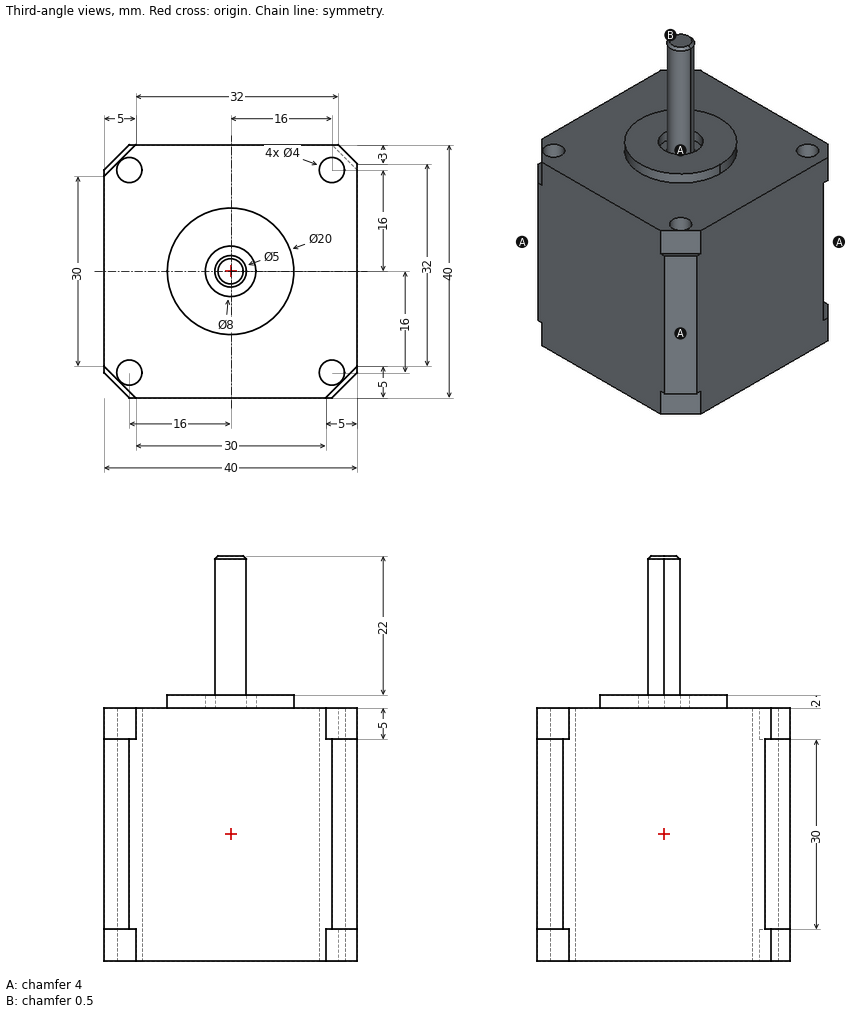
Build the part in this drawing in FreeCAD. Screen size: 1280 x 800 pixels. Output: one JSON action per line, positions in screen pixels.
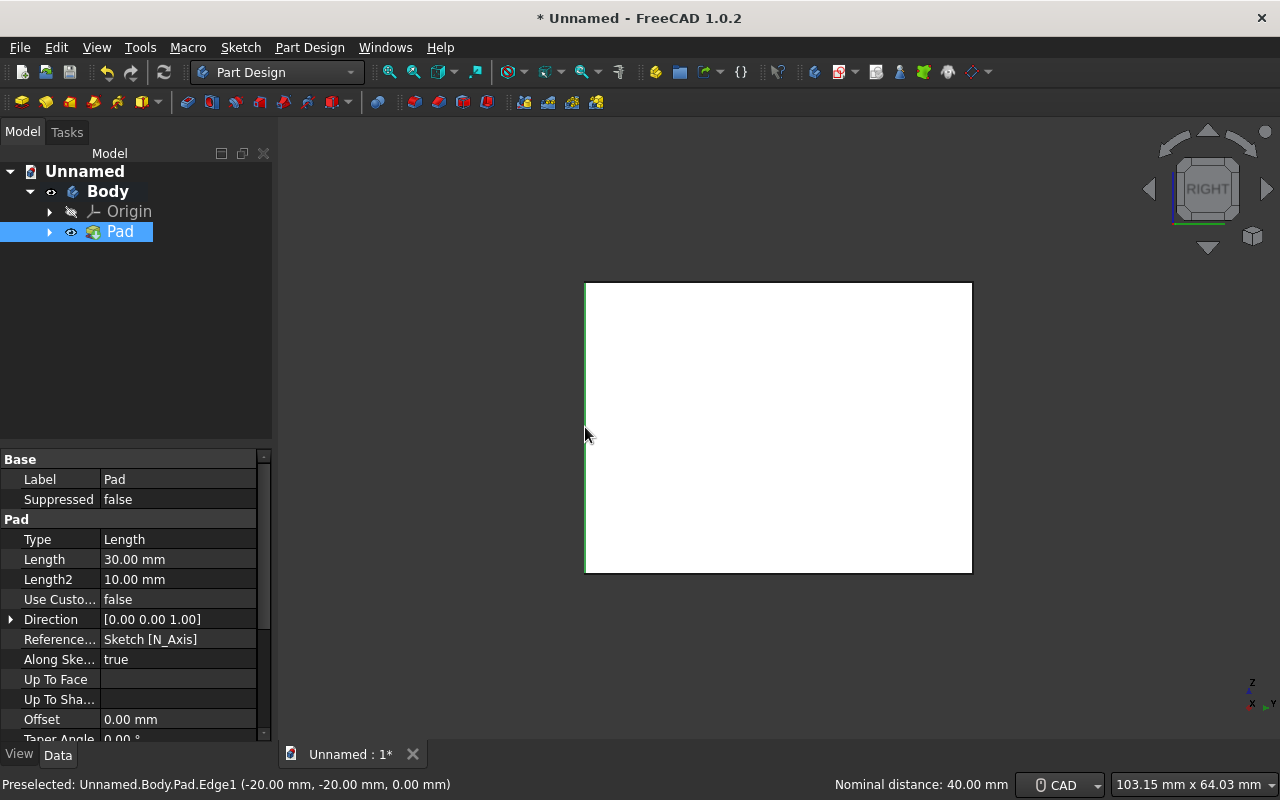
{"action": "left_click", "coordinate": [973, 427], "text": "ctrl"}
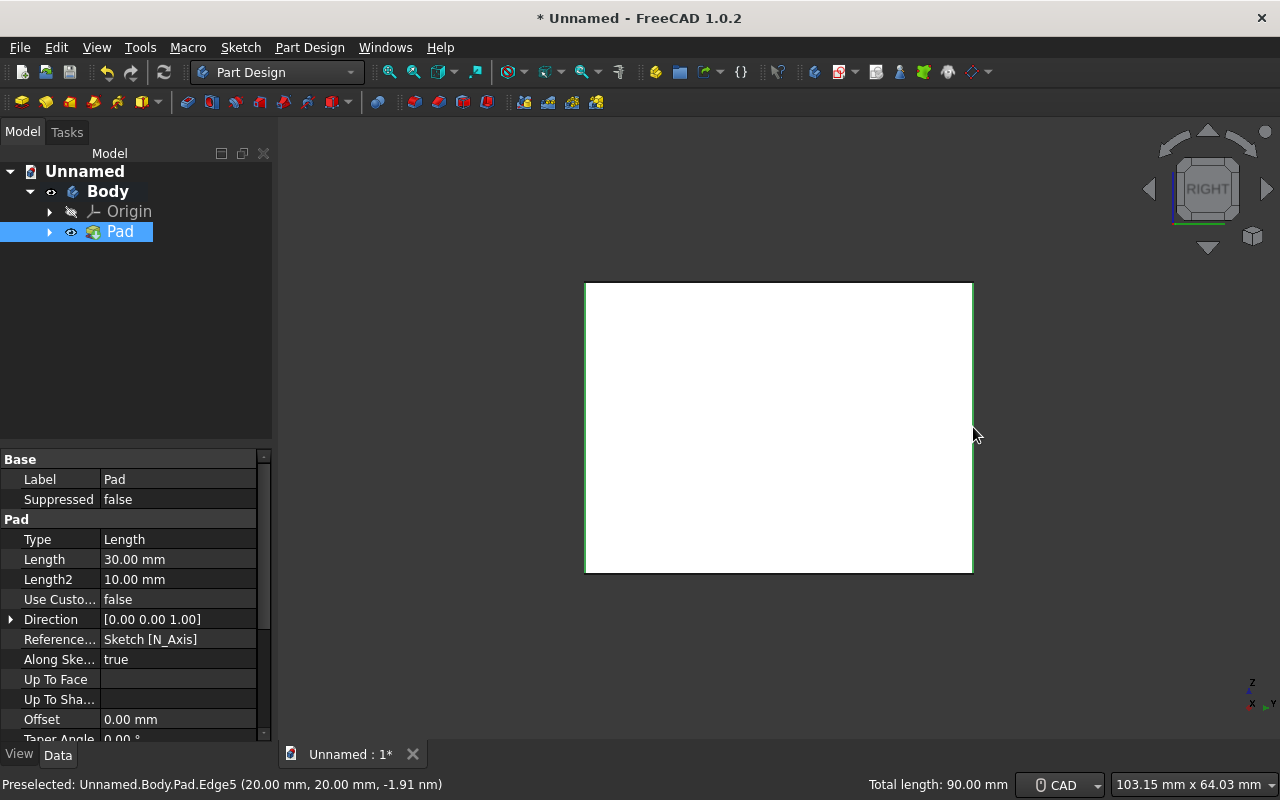
{"action": "key", "text": "5"}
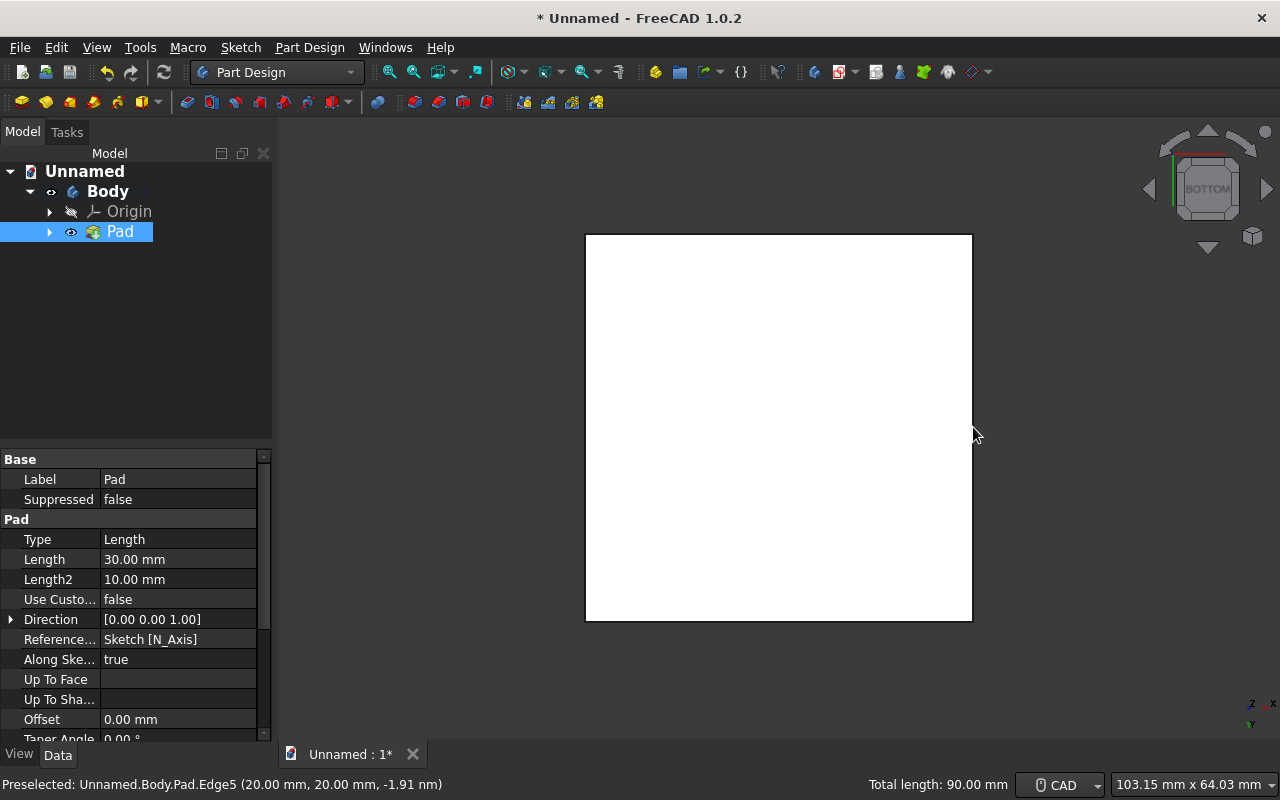
{"action": "key", "text": "4"}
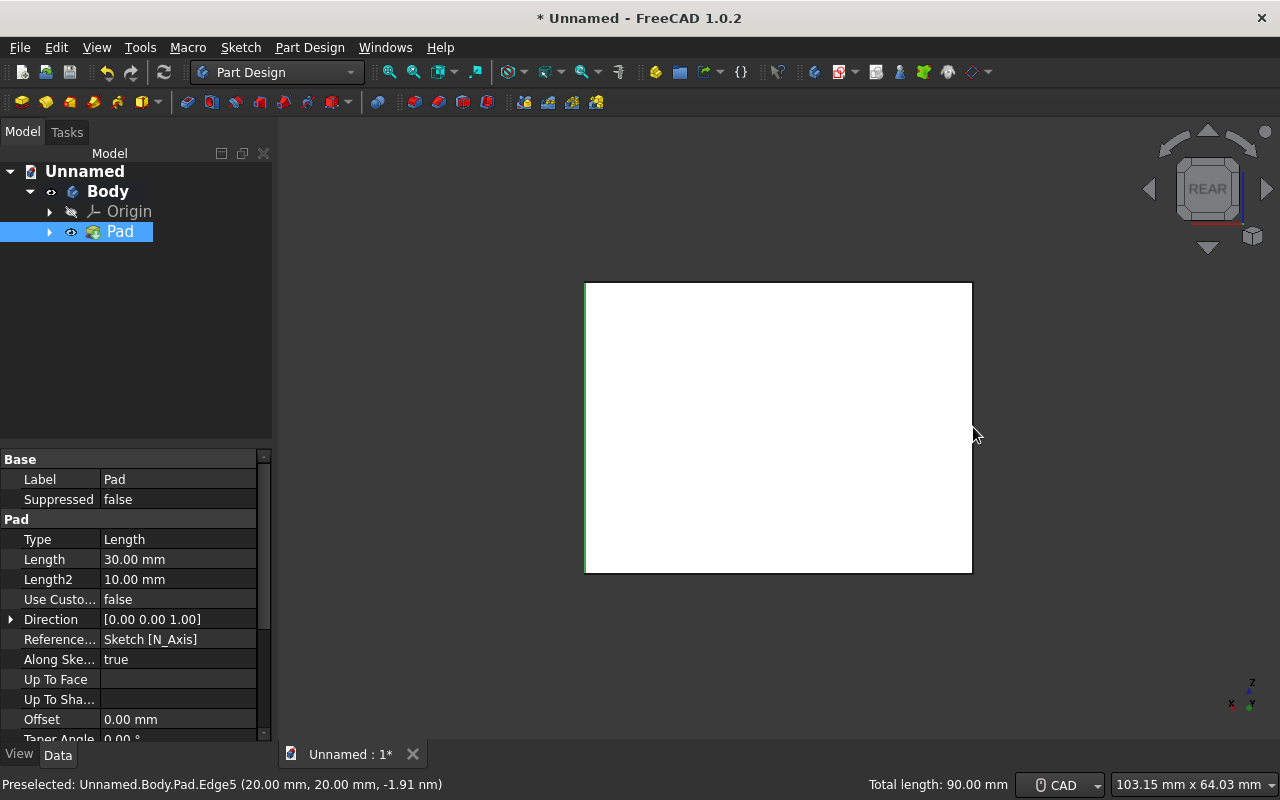
{"action": "left_click", "coordinate": [973, 427], "text": "ctrl"}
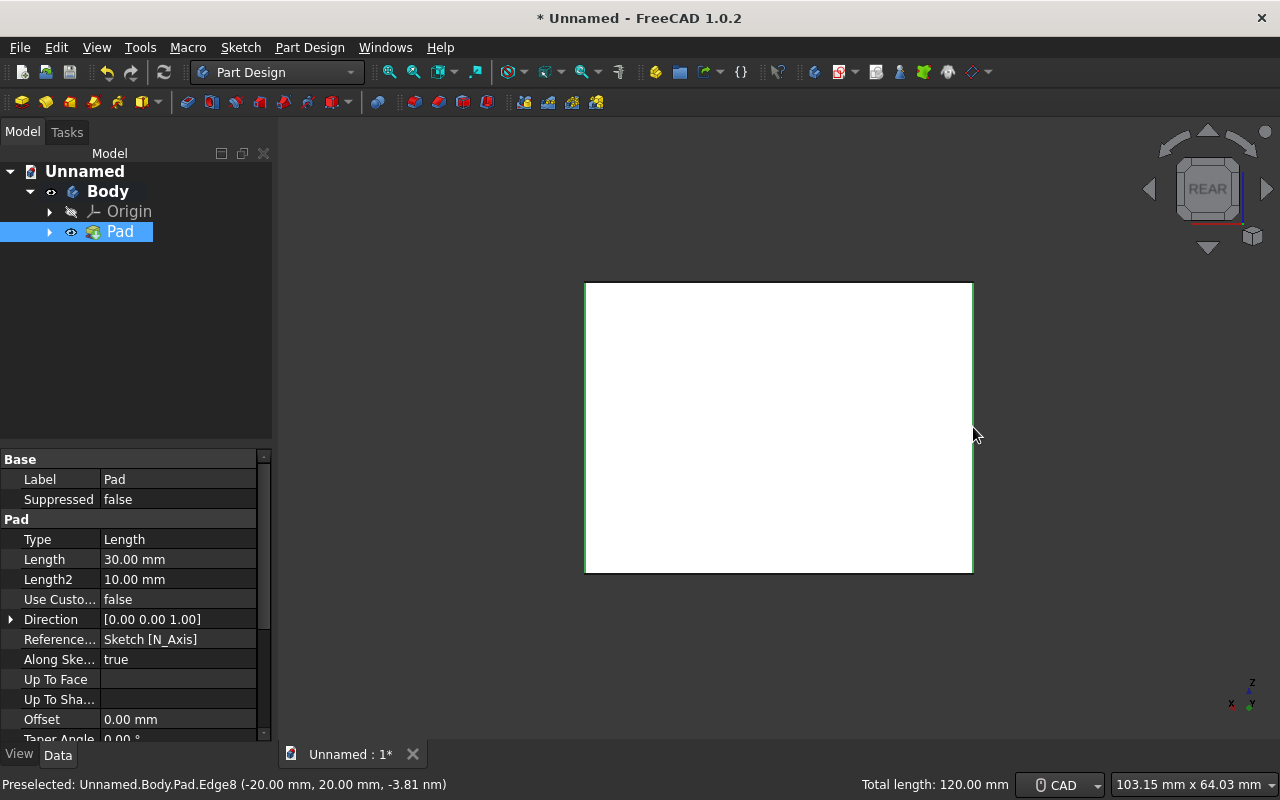
{"action": "left_click", "coordinate": [440, 102]}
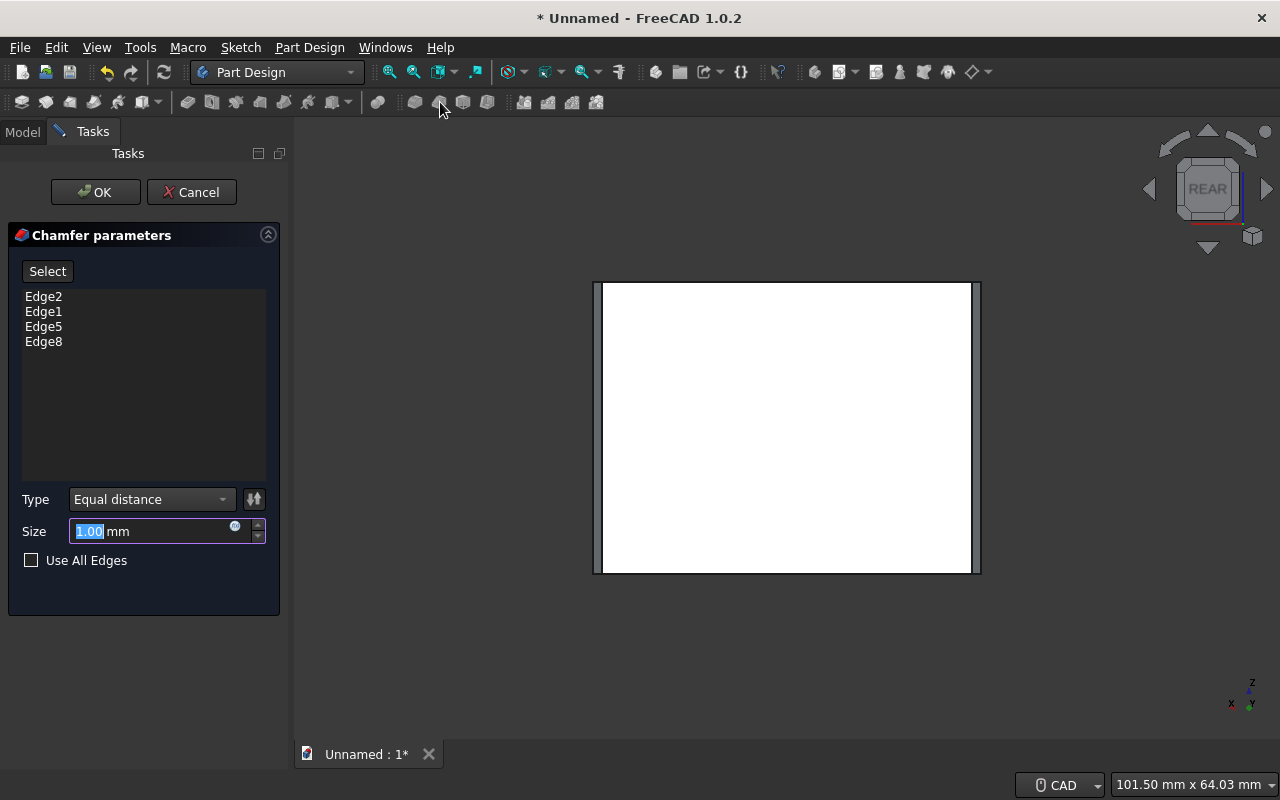
{"action": "type", "text": "4"}
{"action": "key", "text": "Tab"}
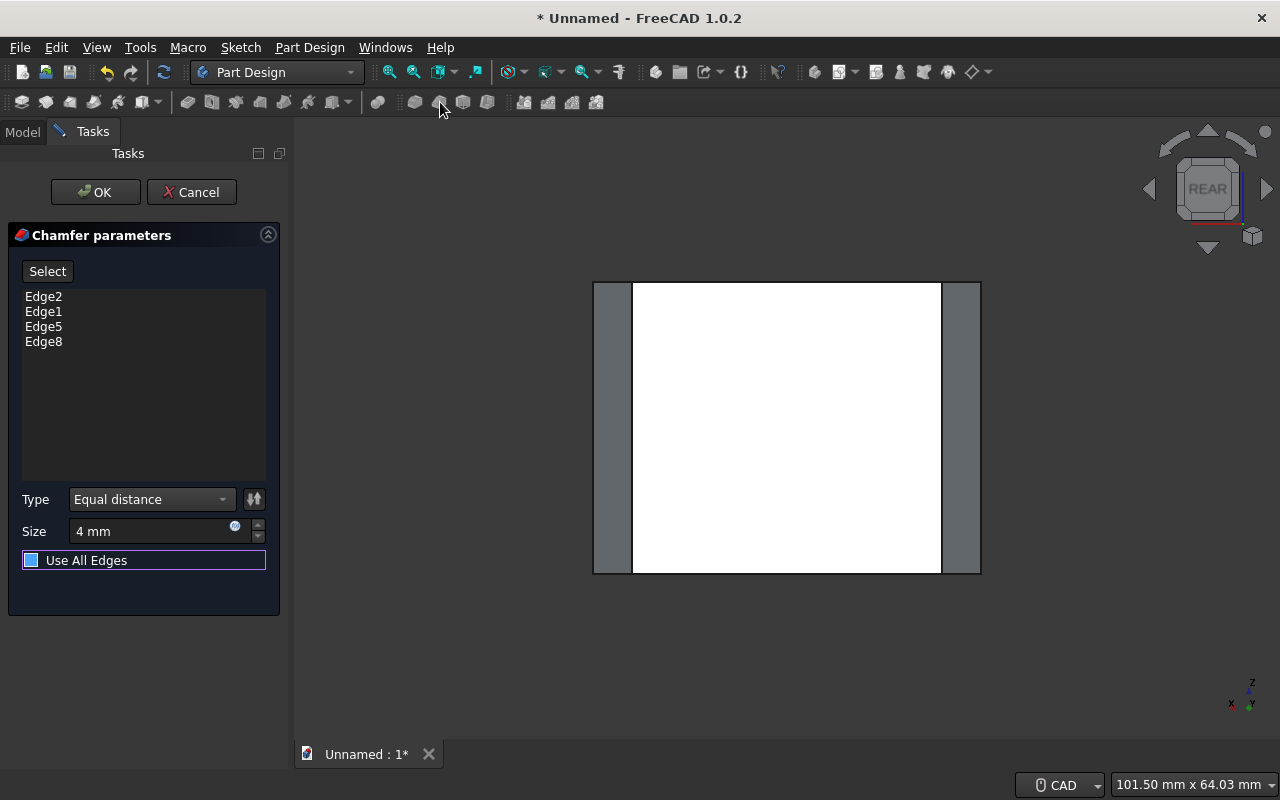
{"action": "left_click", "coordinate": [96, 192]}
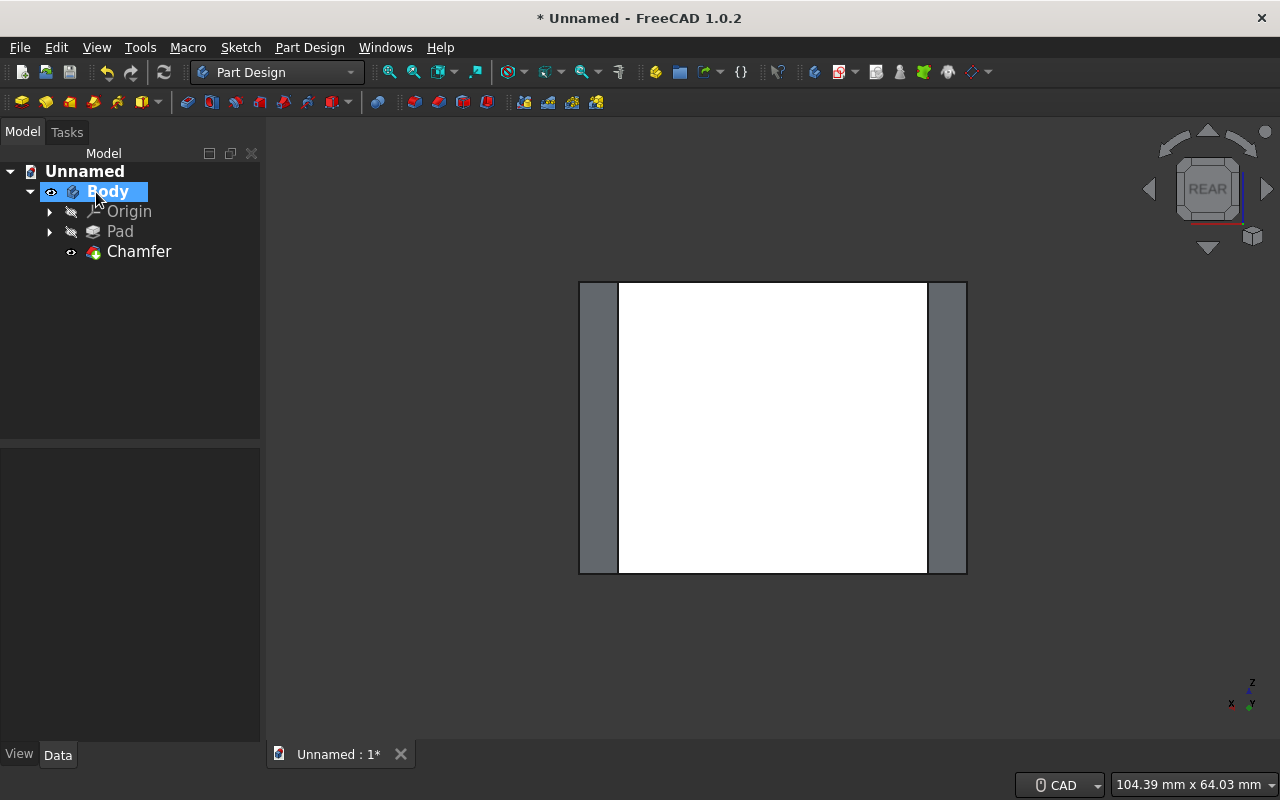
{"action": "key", "text": "0"}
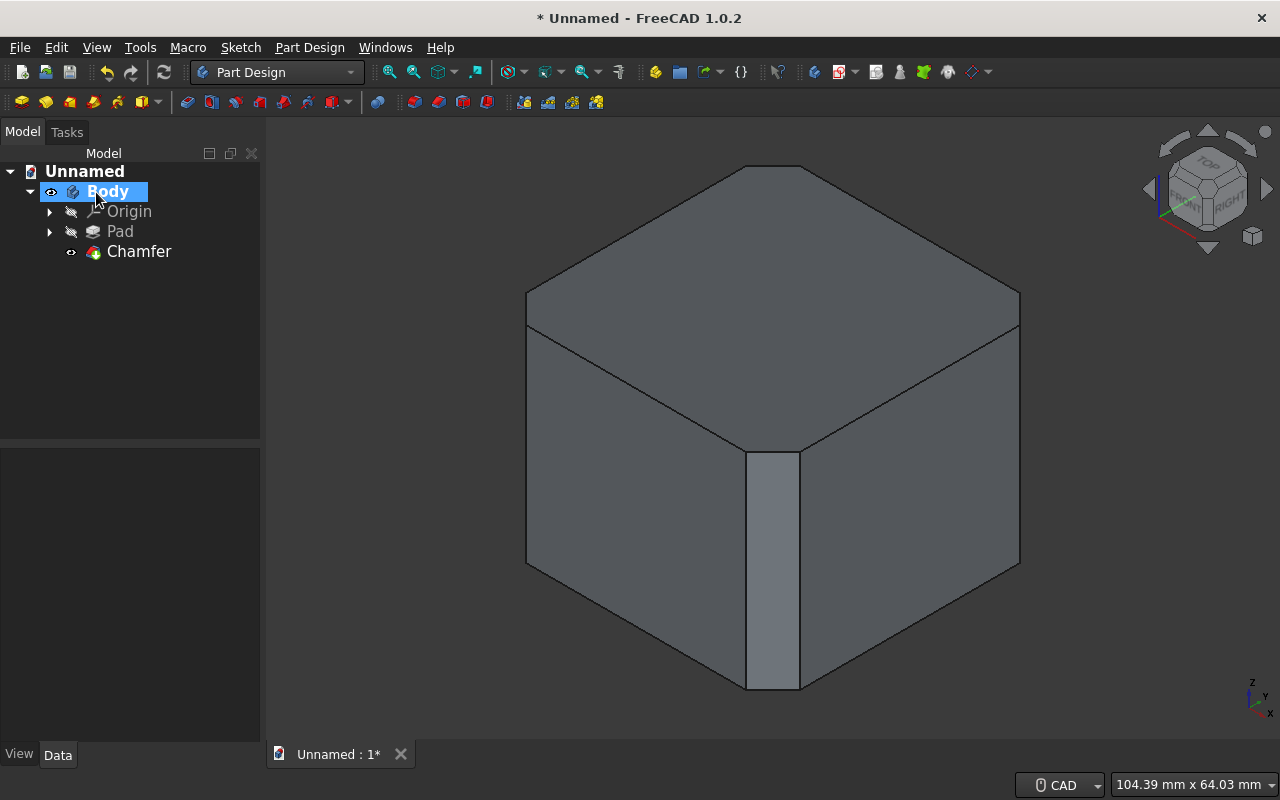
{"action": "left_click", "coordinate": [773, 308]}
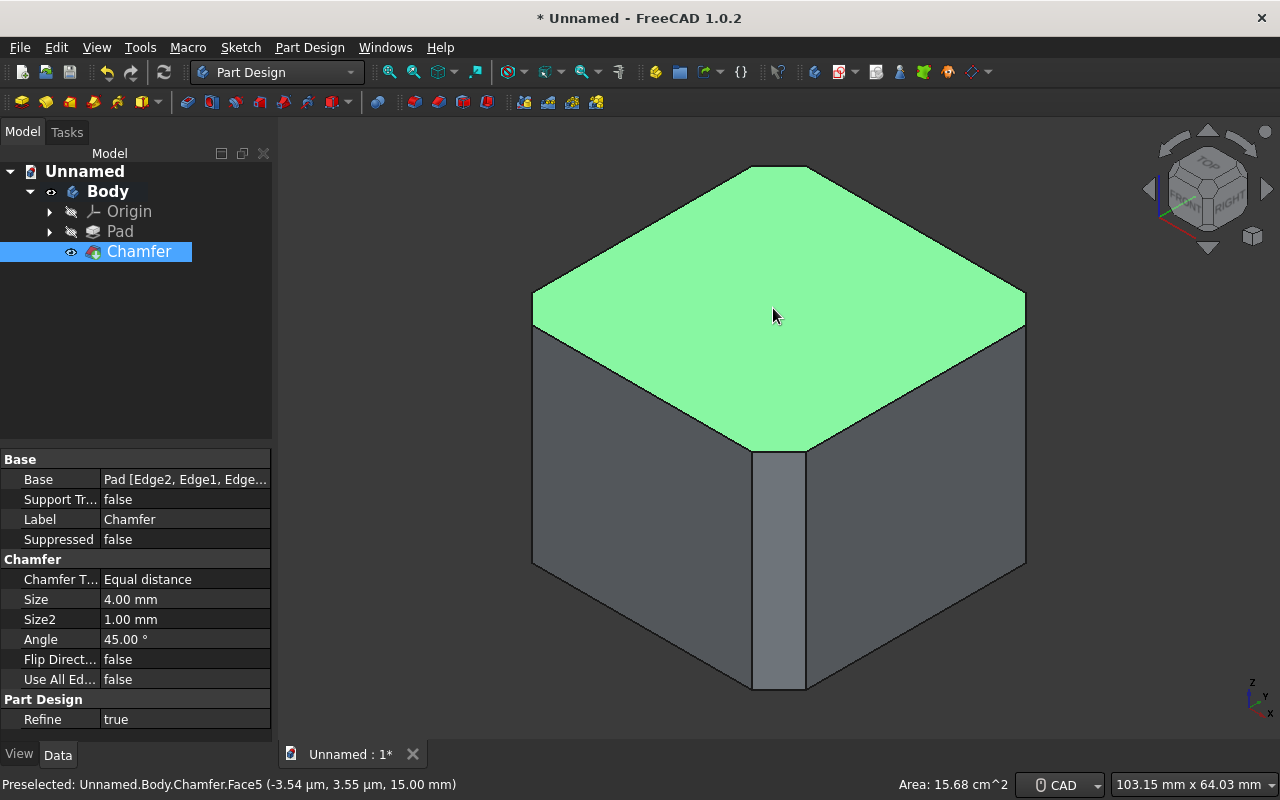
{"action": "left_click", "coordinate": [840, 72]}